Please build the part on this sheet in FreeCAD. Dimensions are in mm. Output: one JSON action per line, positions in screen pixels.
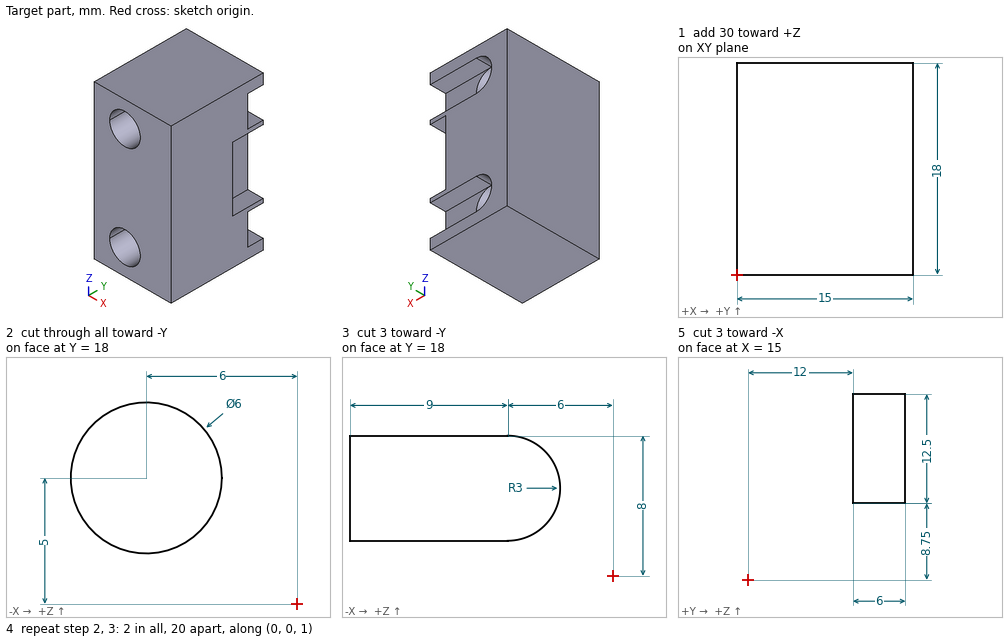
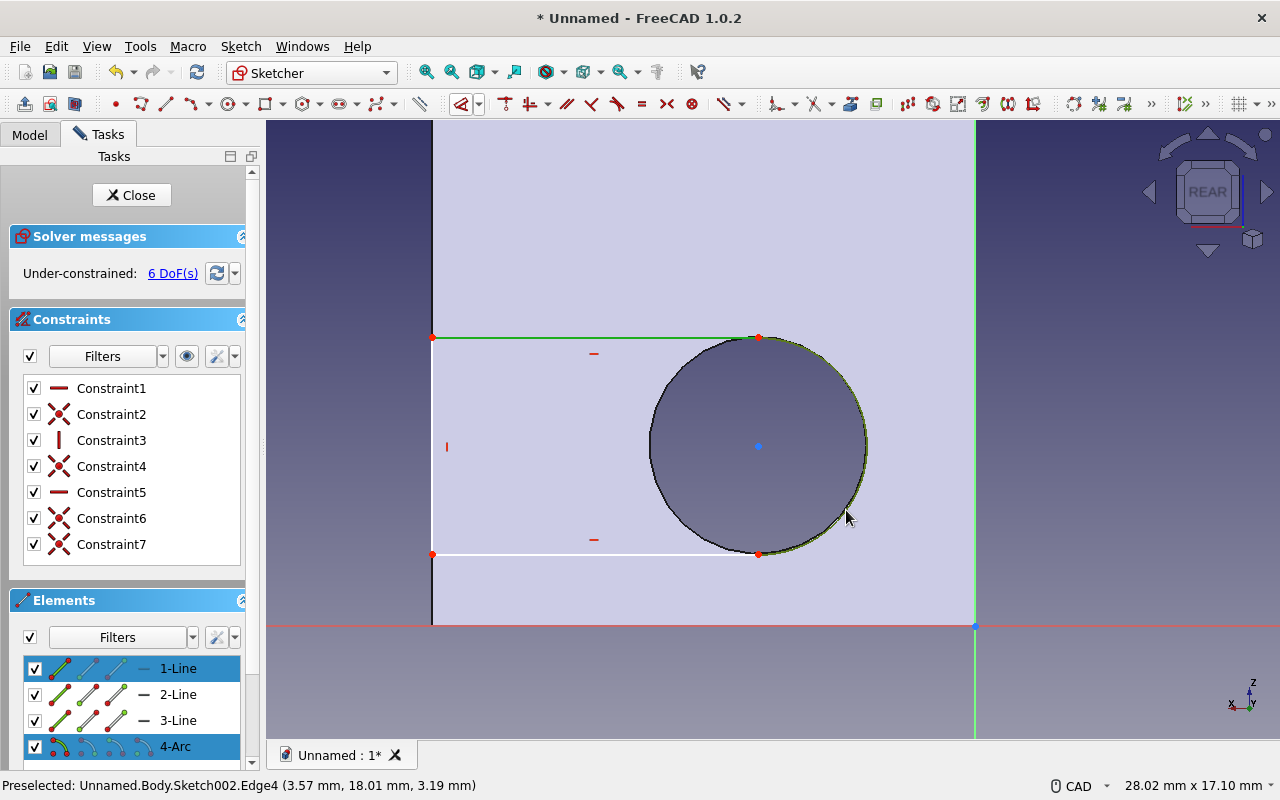
{"action": "left_click", "coordinate": [617, 104]}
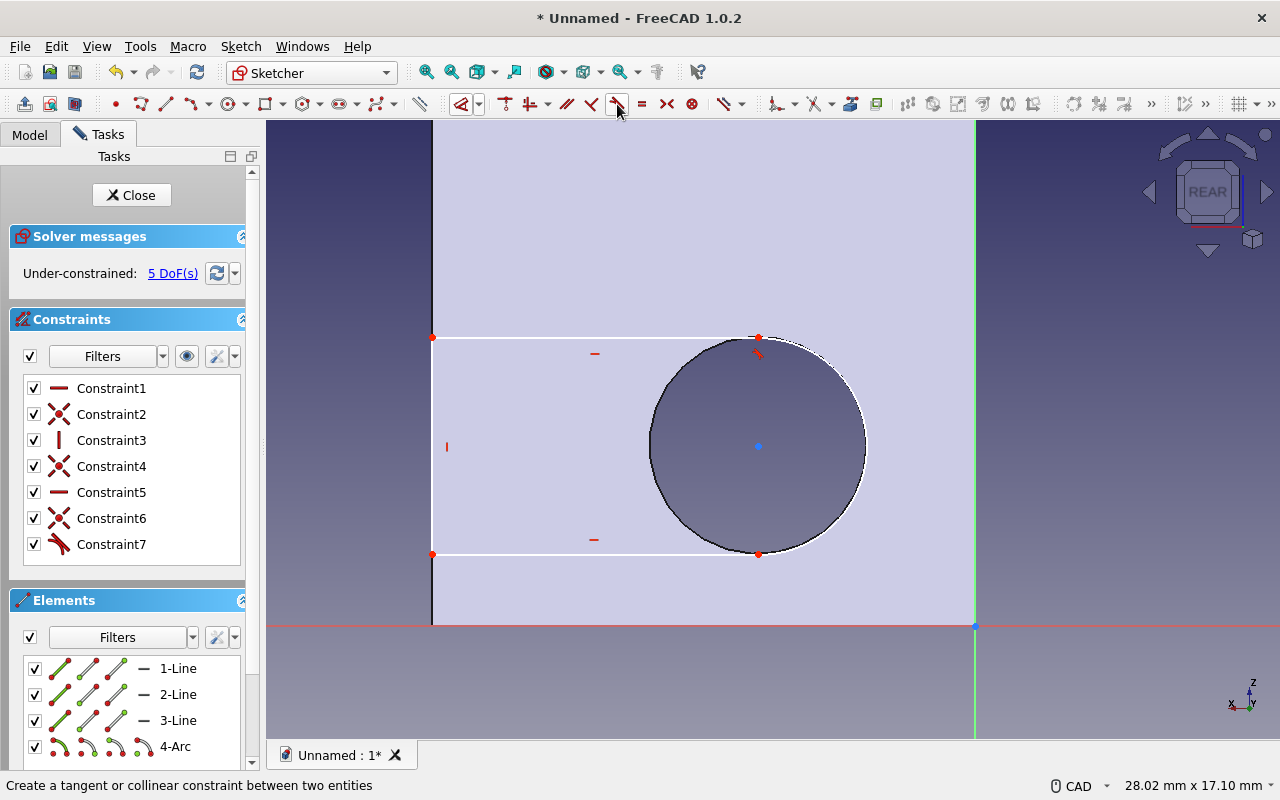
{"action": "left_click", "coordinate": [530, 555]}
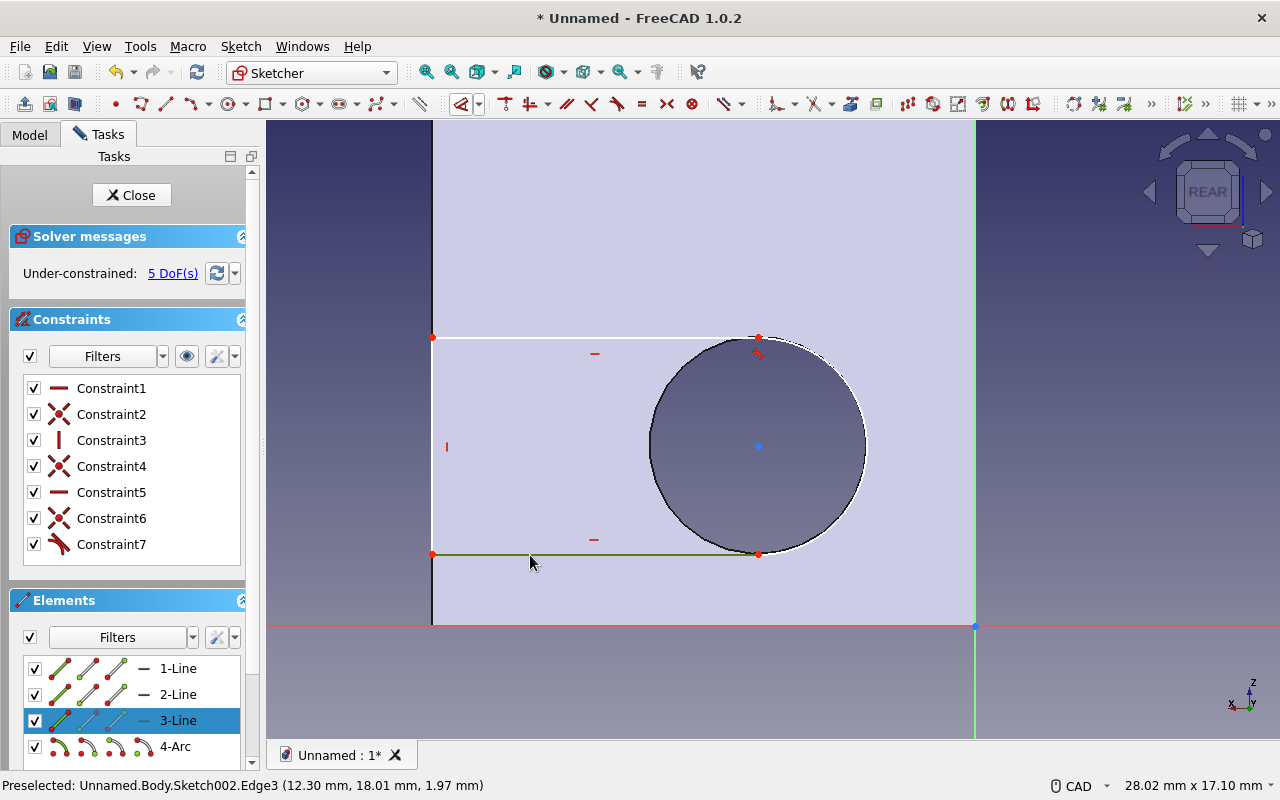
{"action": "left_click", "coordinate": [846, 511]}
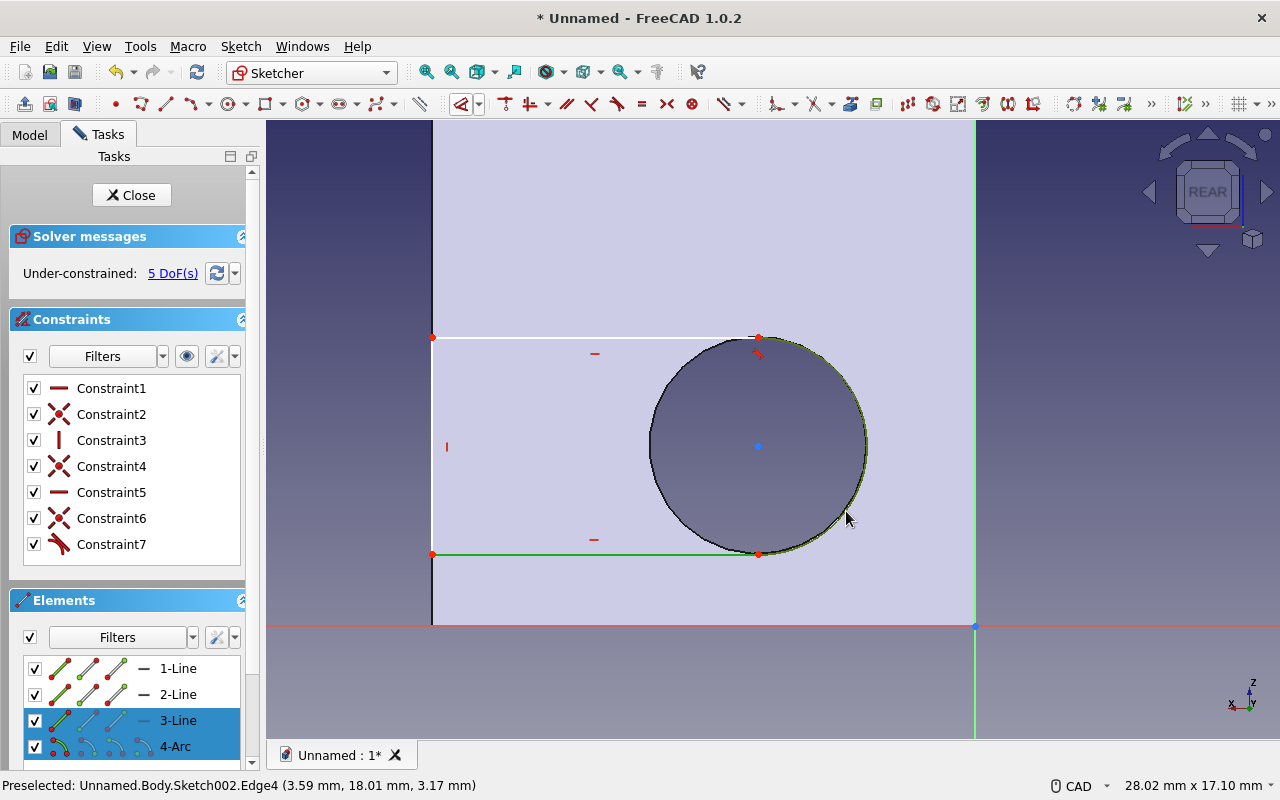
{"action": "left_click", "coordinate": [617, 104]}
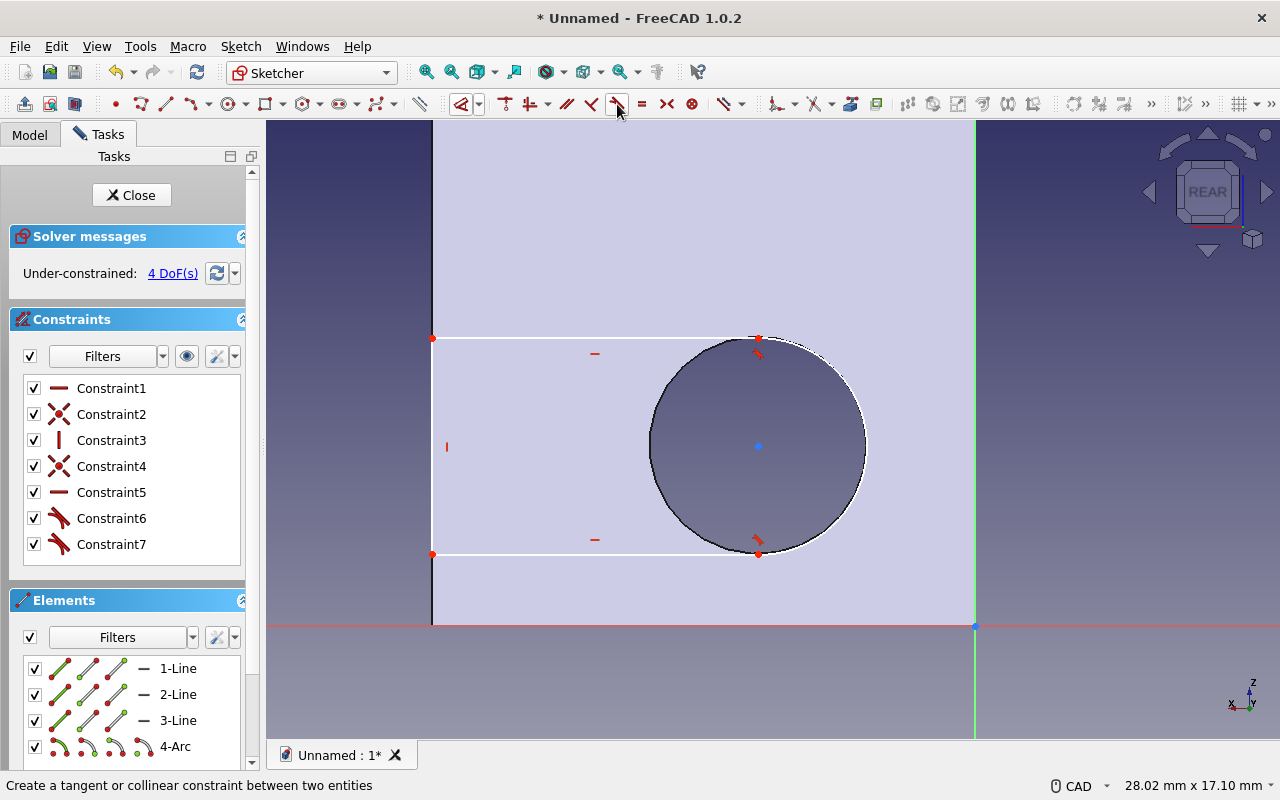
{"action": "left_click", "coordinate": [846, 510]}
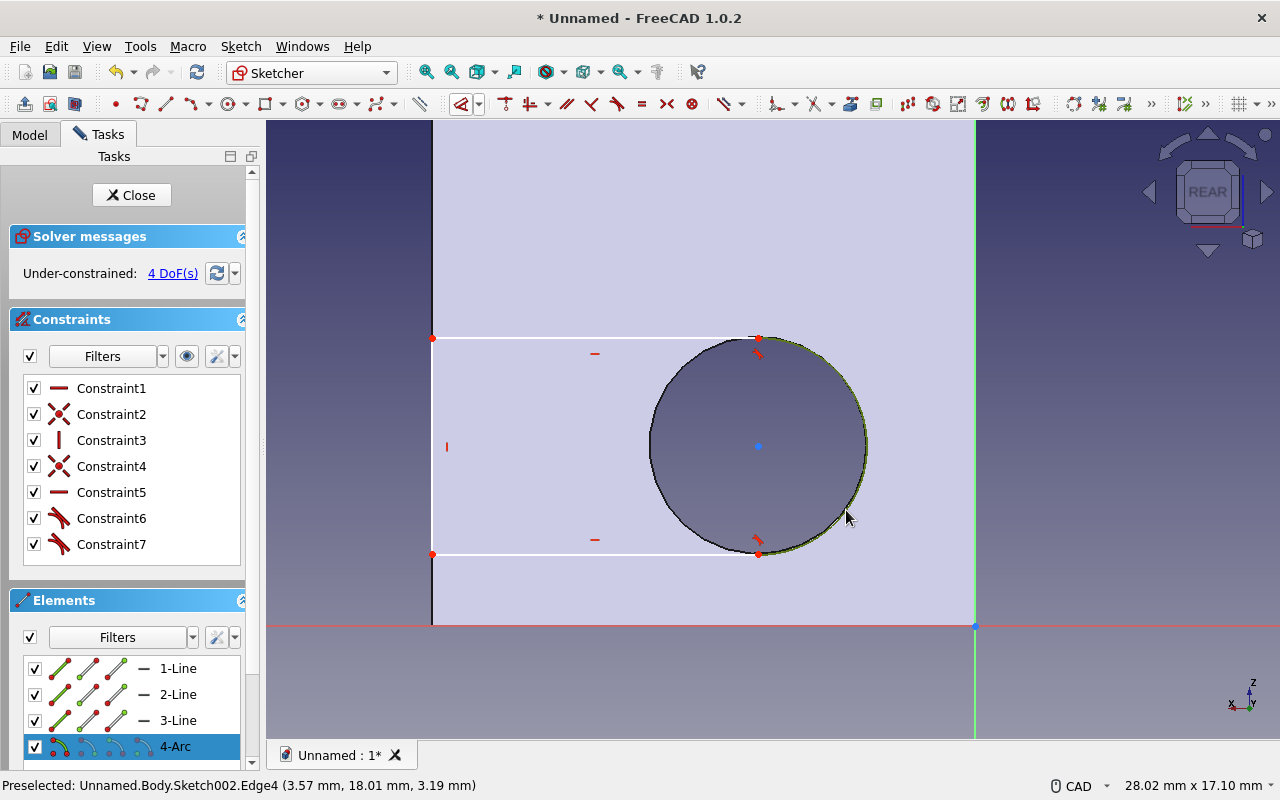
{"action": "key", "text": "k r"}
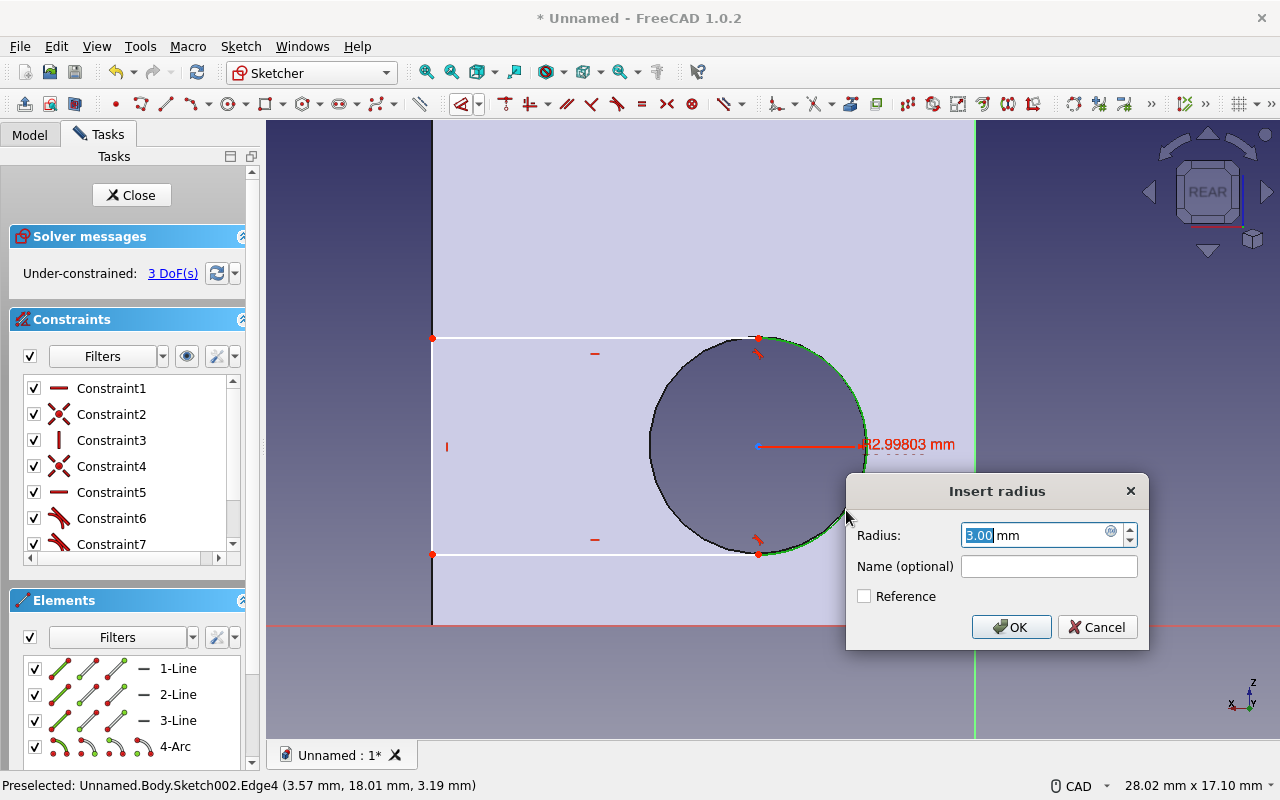
{"action": "type", "text": "3"}
{"action": "key", "text": "Return"}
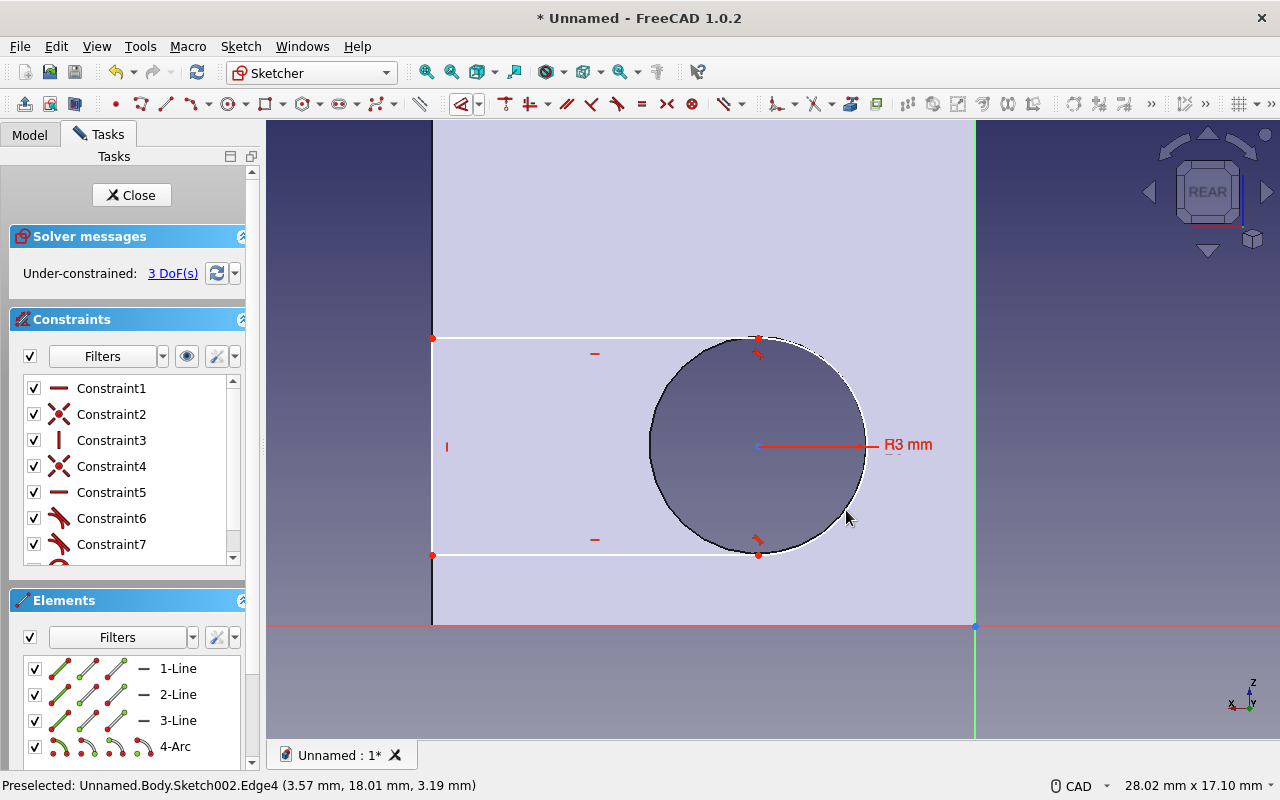
{"action": "left_click", "coordinate": [661, 338]}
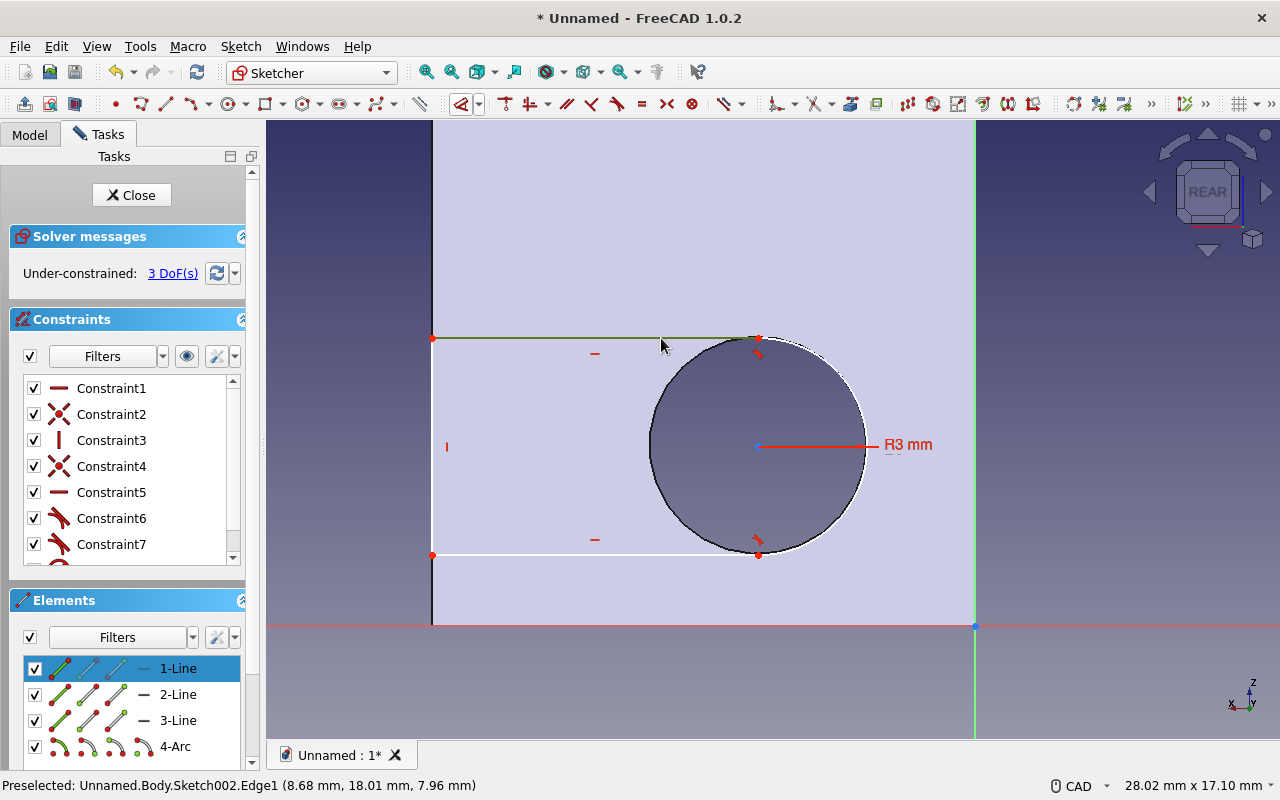
{"action": "key", "text": "l"}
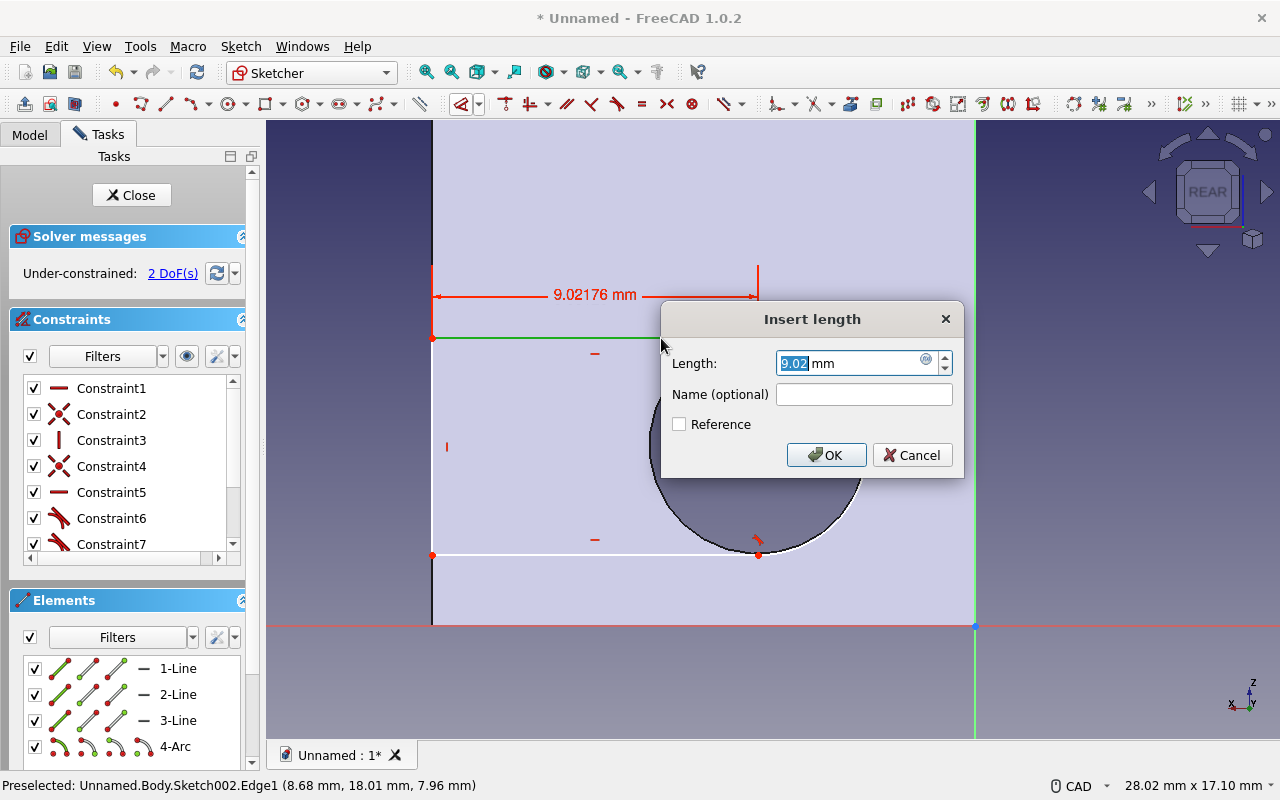
{"action": "type", "text": "9"}
{"action": "key", "text": "Return"}